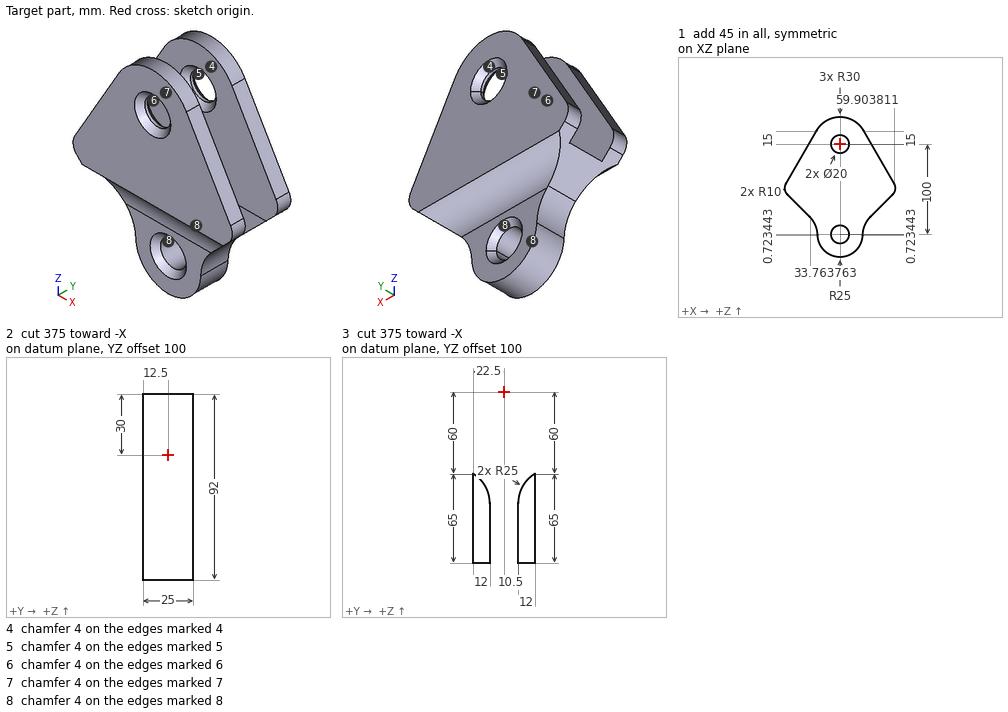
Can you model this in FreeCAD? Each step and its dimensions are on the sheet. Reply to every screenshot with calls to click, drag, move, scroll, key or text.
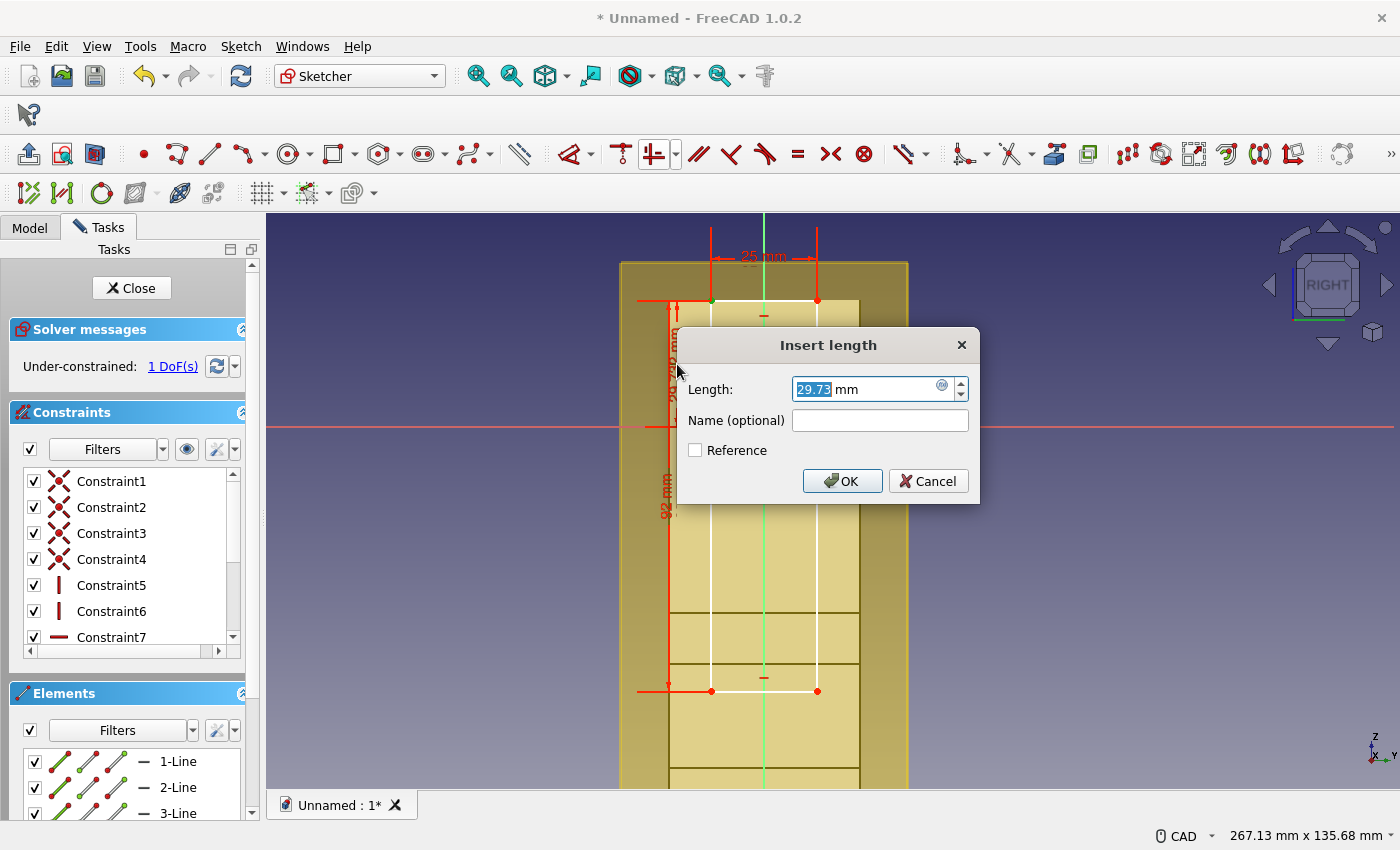
text(30)
key(Return)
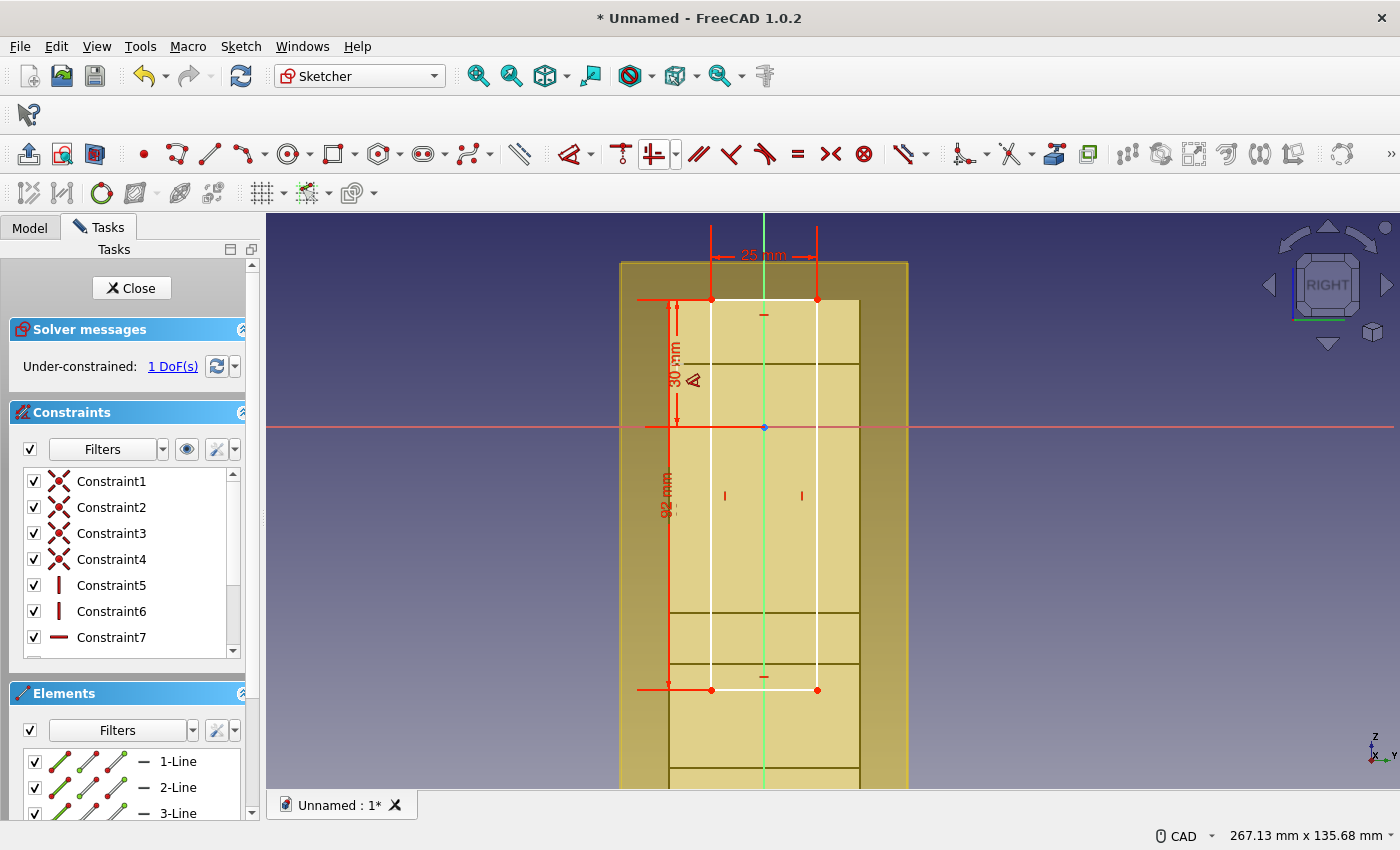
click(711, 300)
click(738, 266)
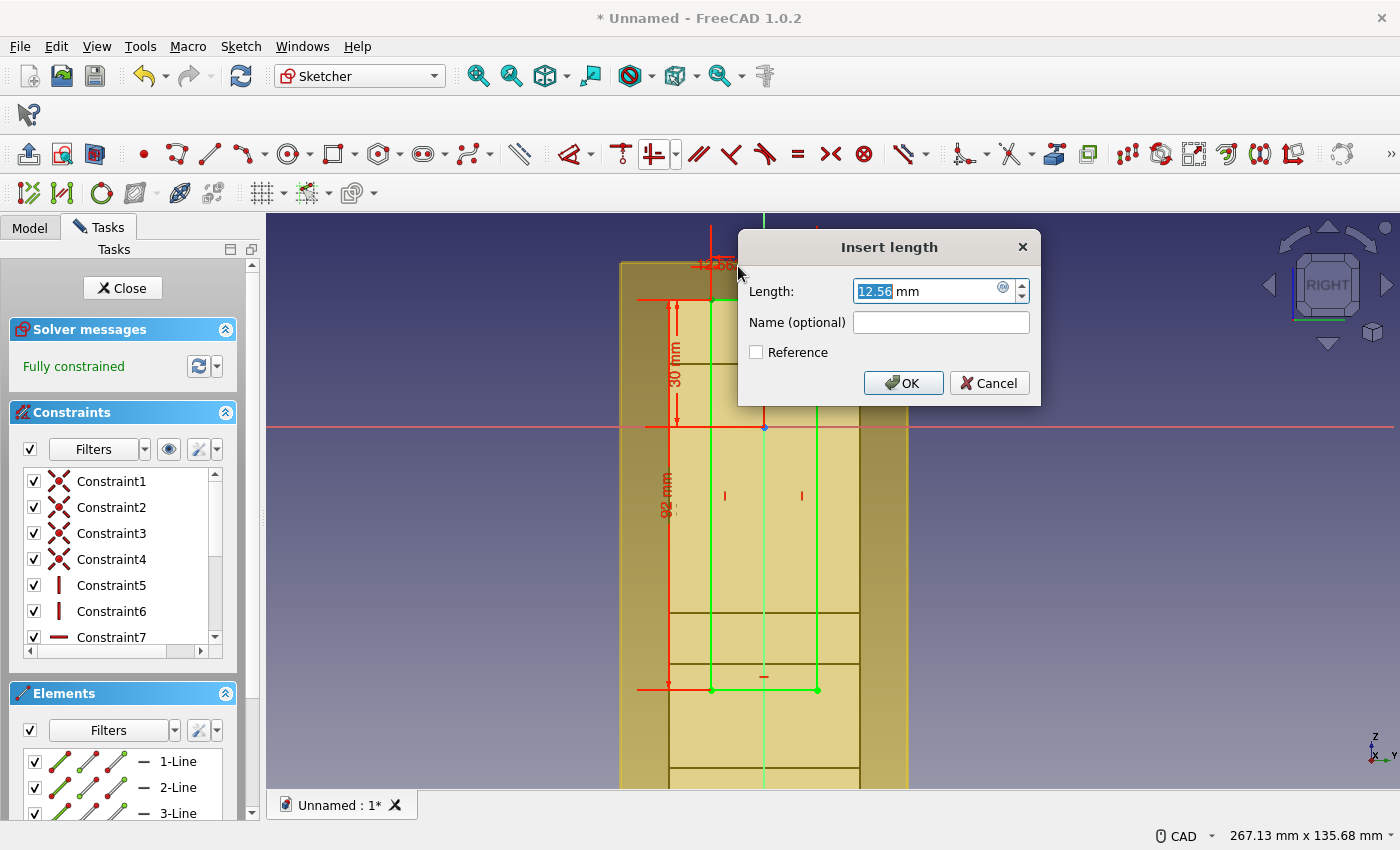
text(12.5)
key(Return)
key(Escape)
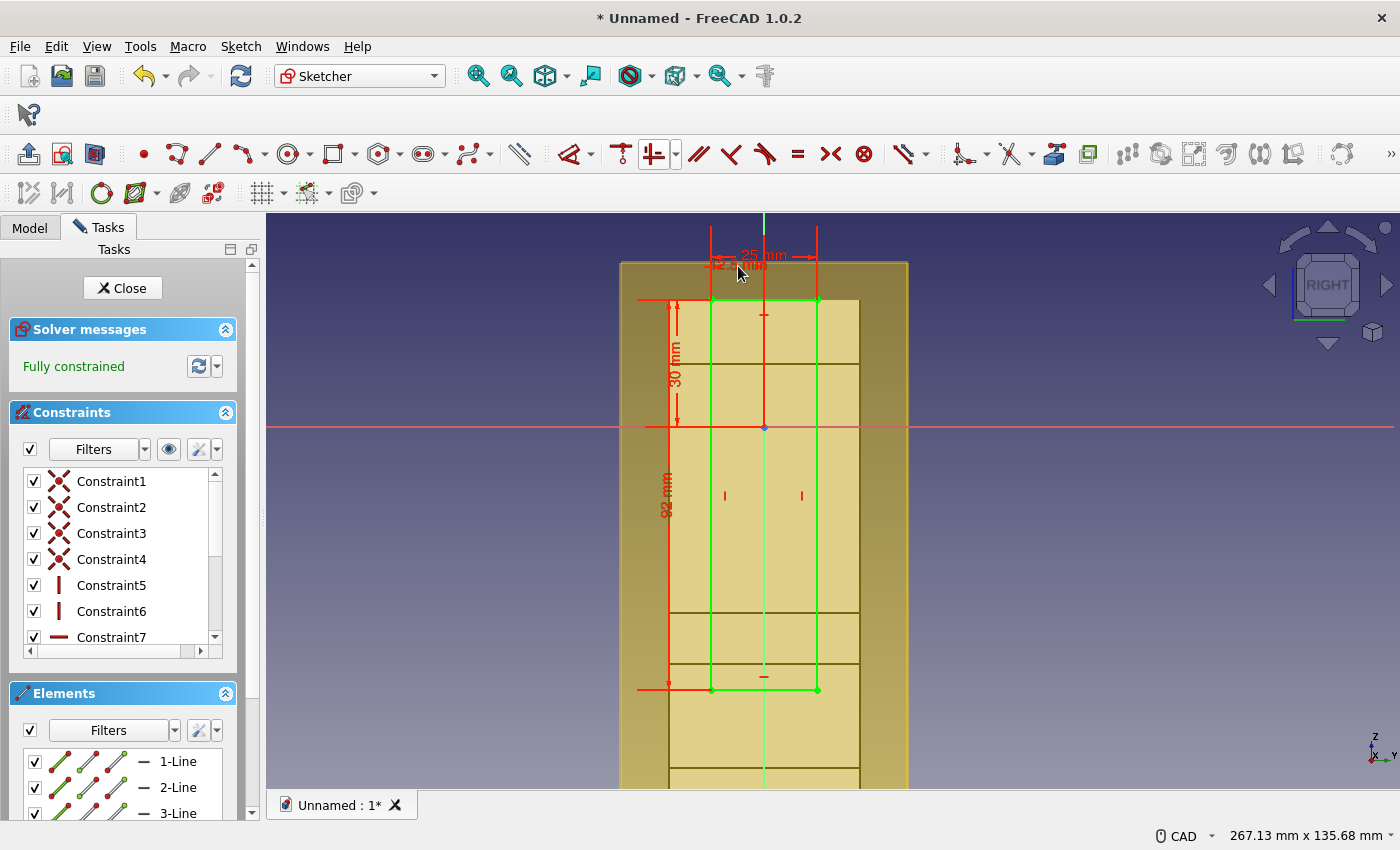
click(123, 288)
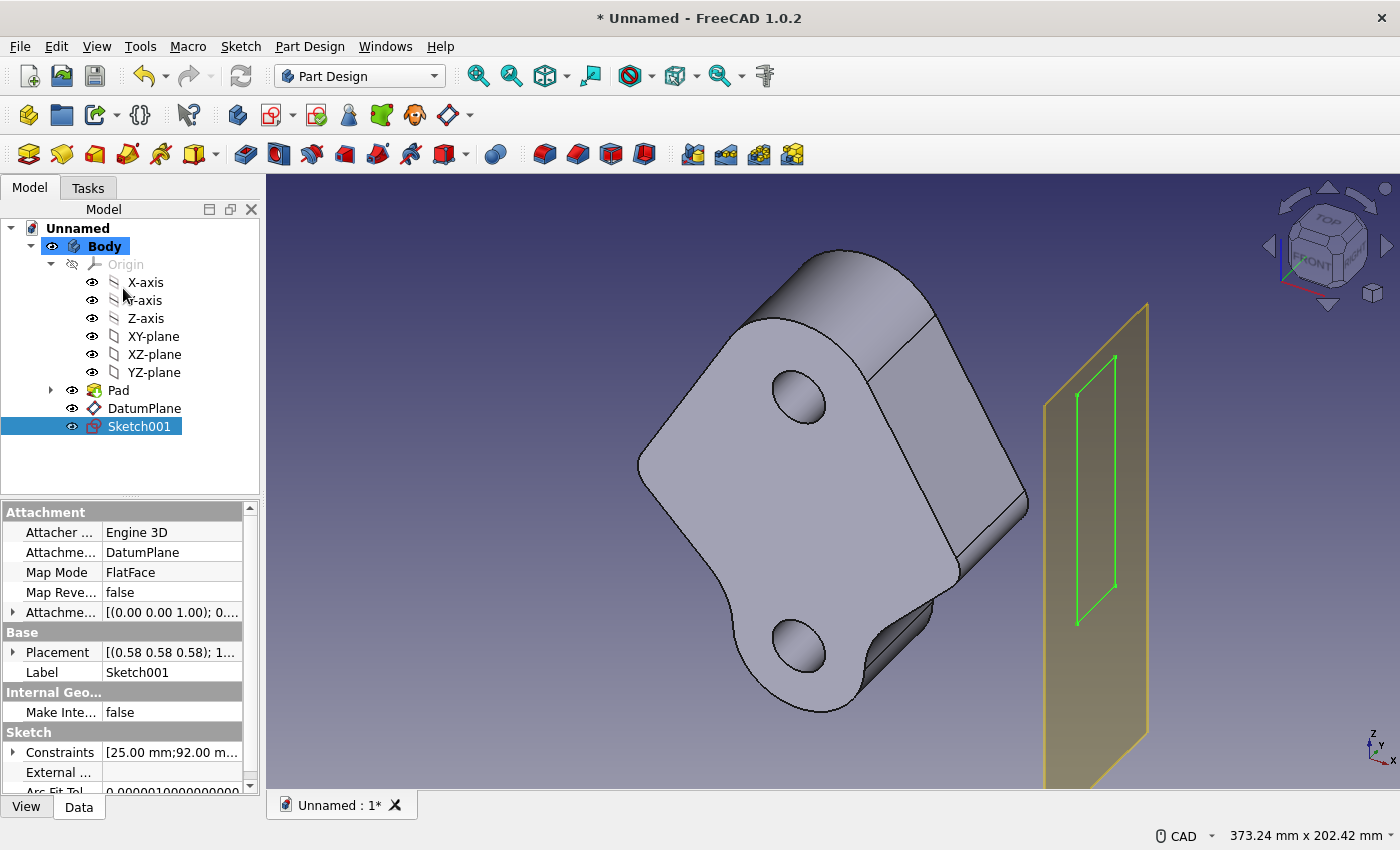
click(246, 154)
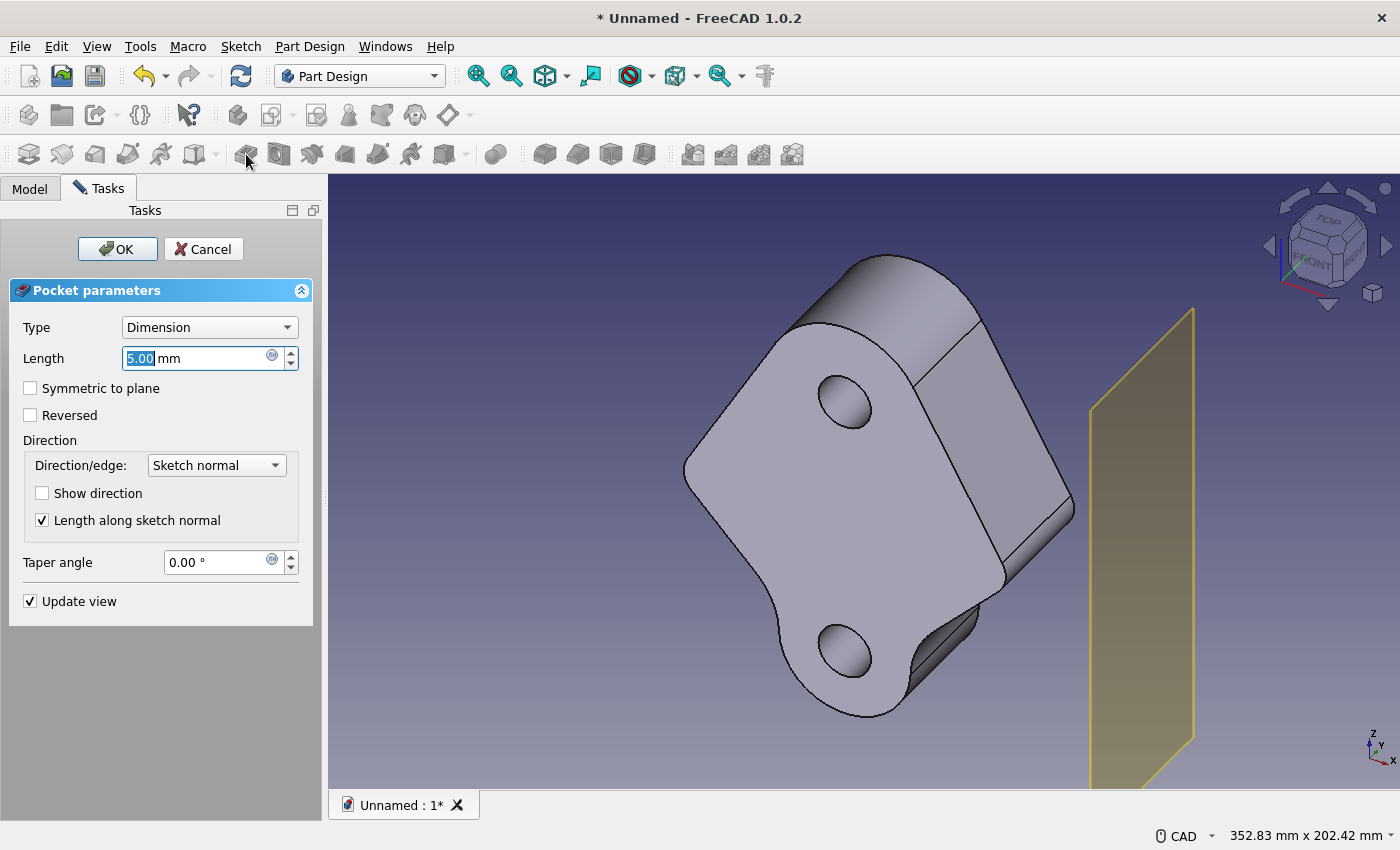
text(375)
key(Tab)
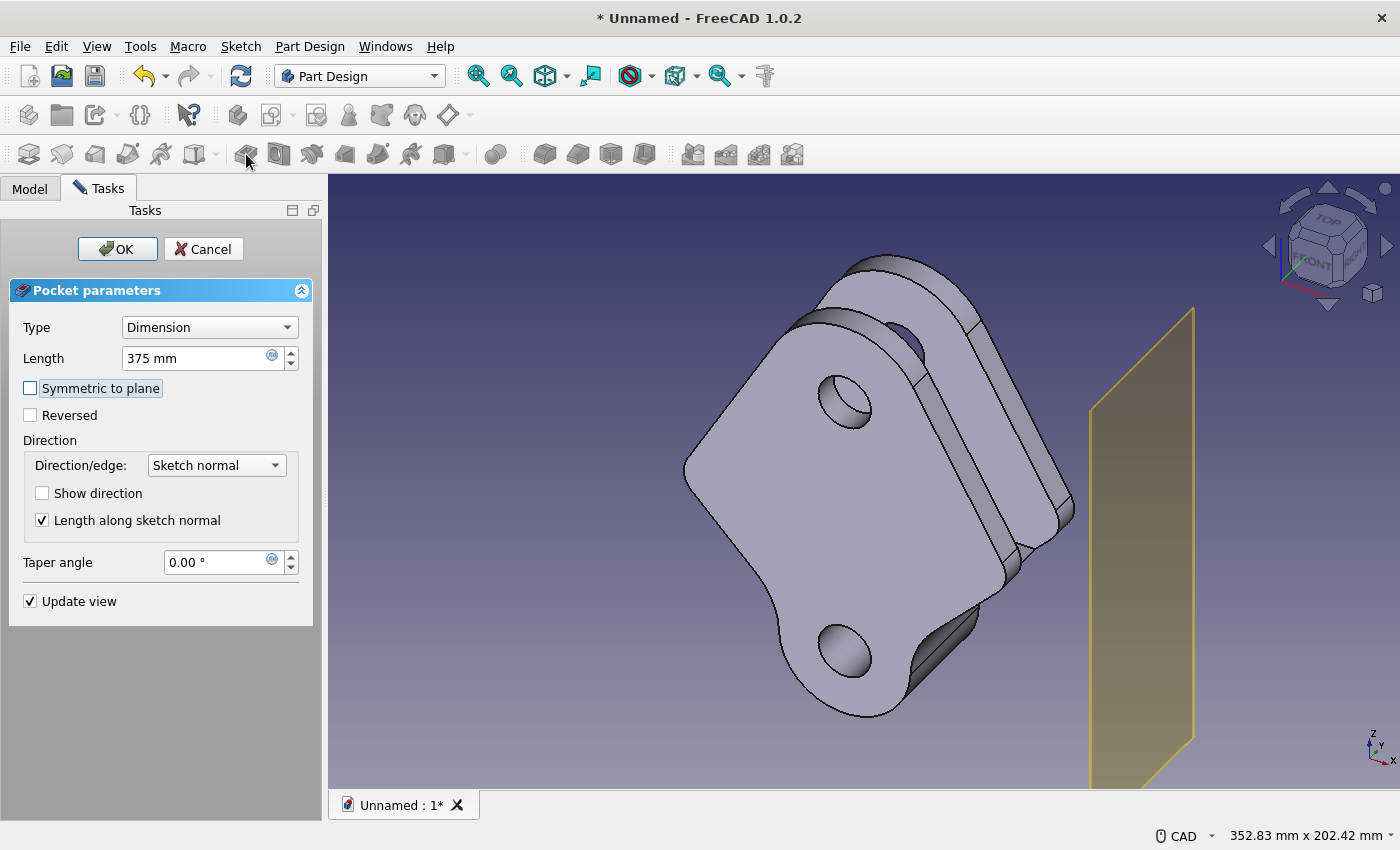
click(118, 249)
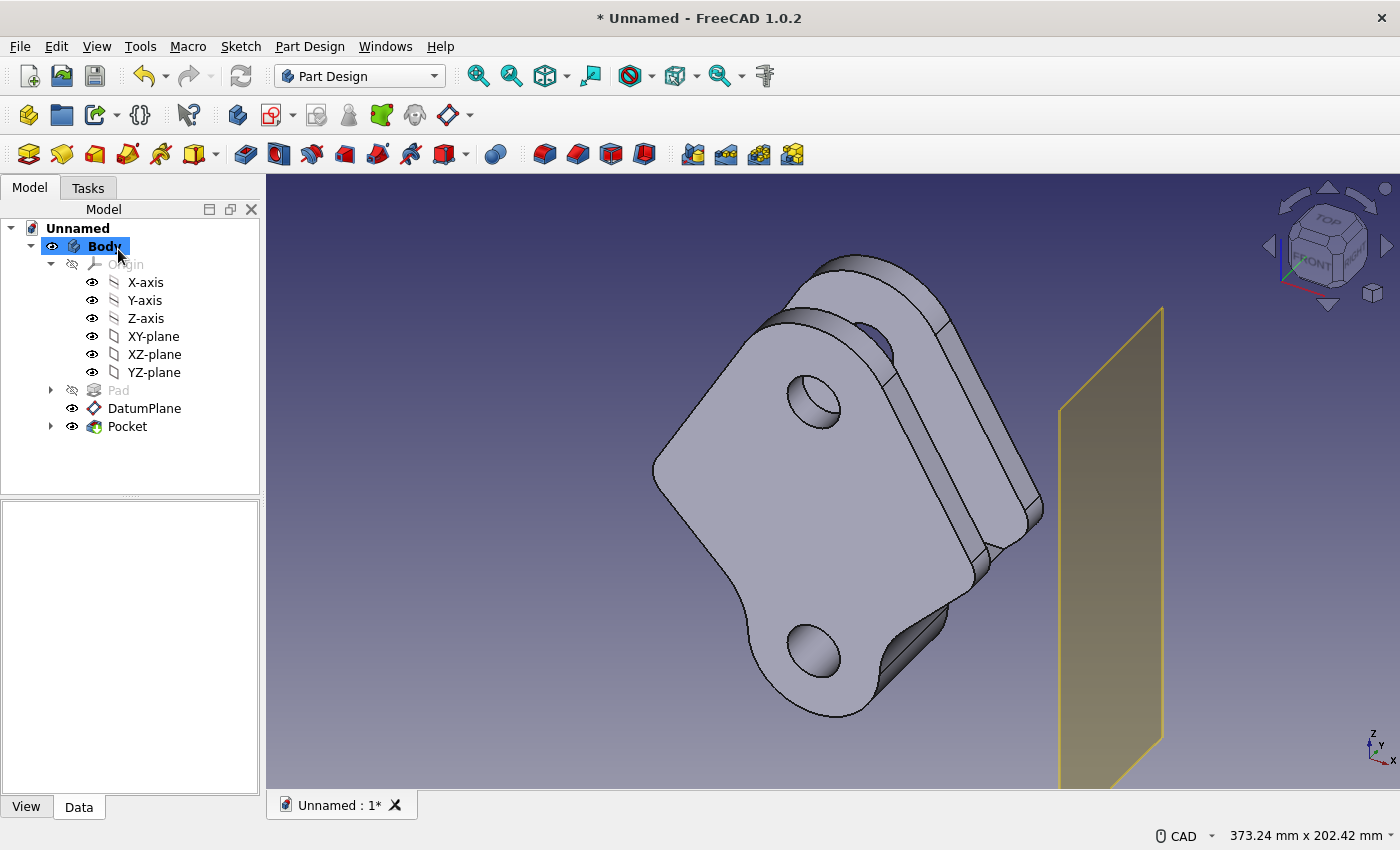
click(117, 408)
key(space)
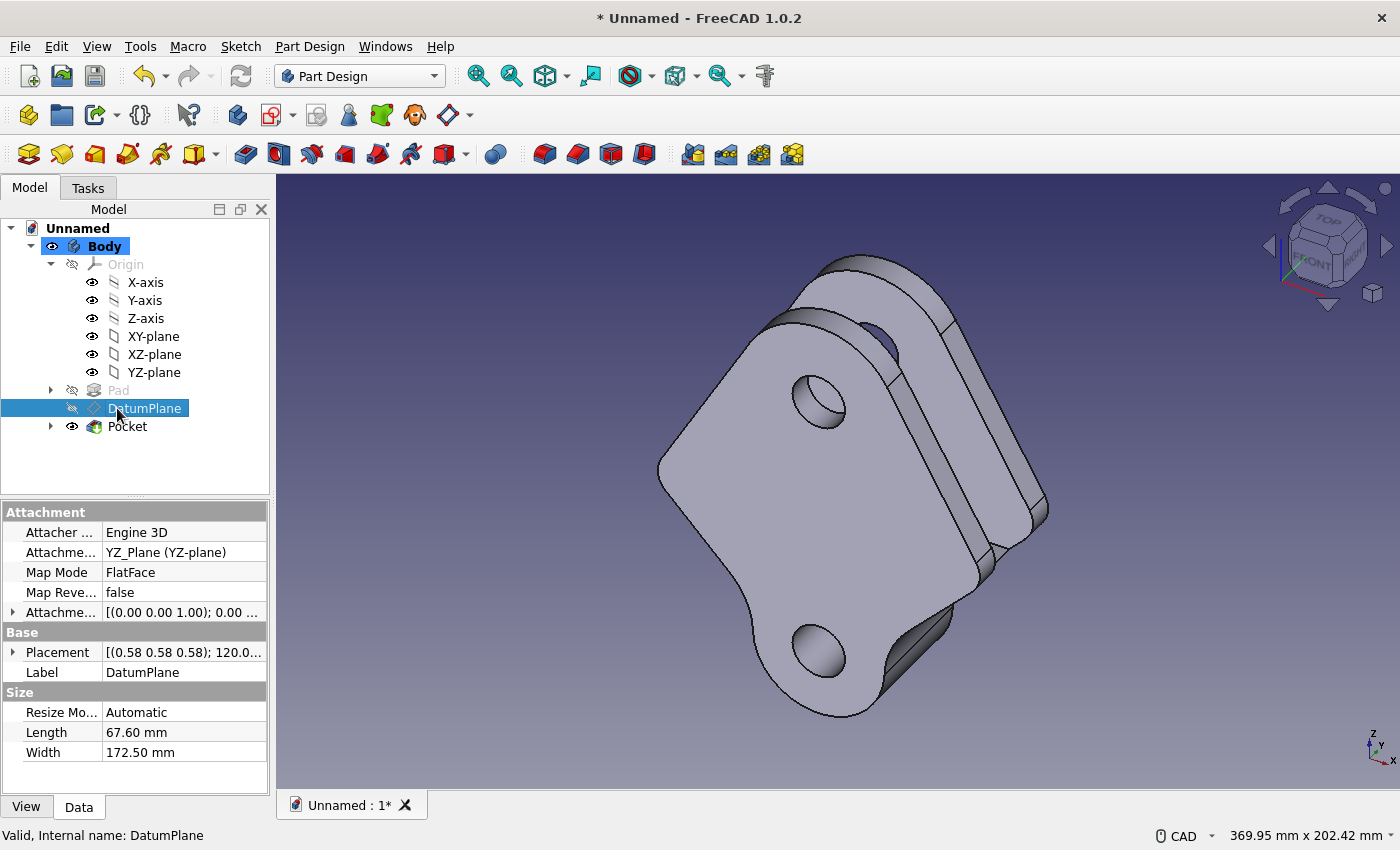
click(137, 372)